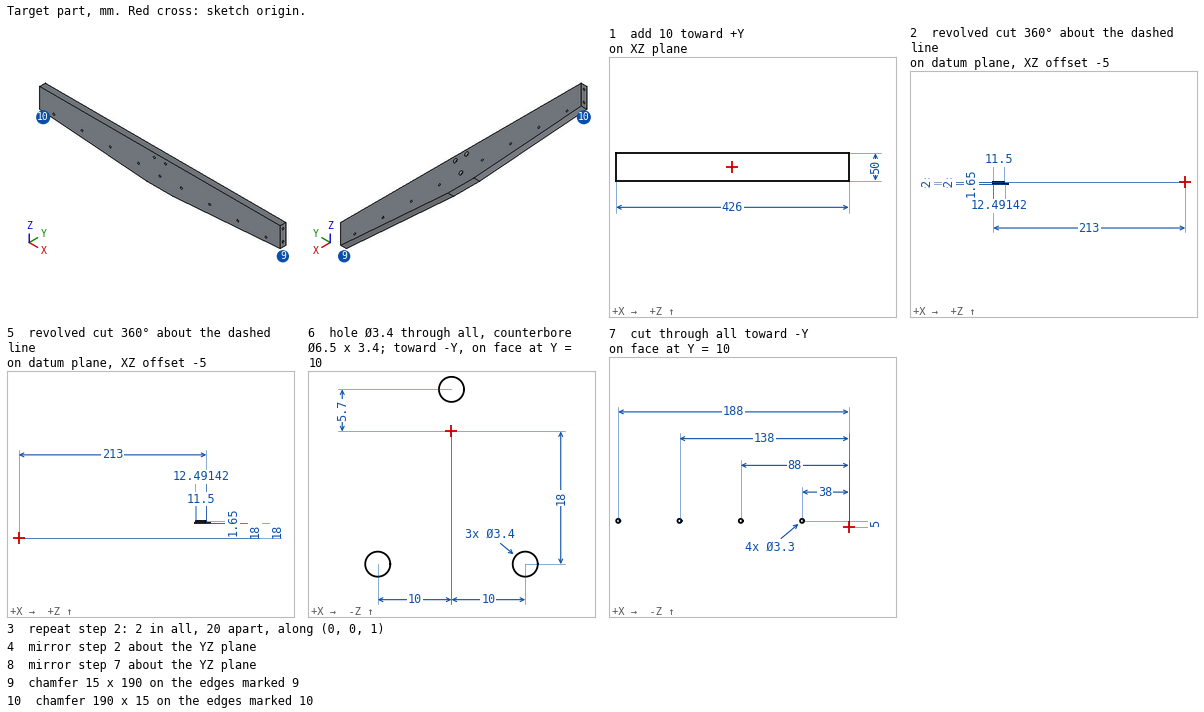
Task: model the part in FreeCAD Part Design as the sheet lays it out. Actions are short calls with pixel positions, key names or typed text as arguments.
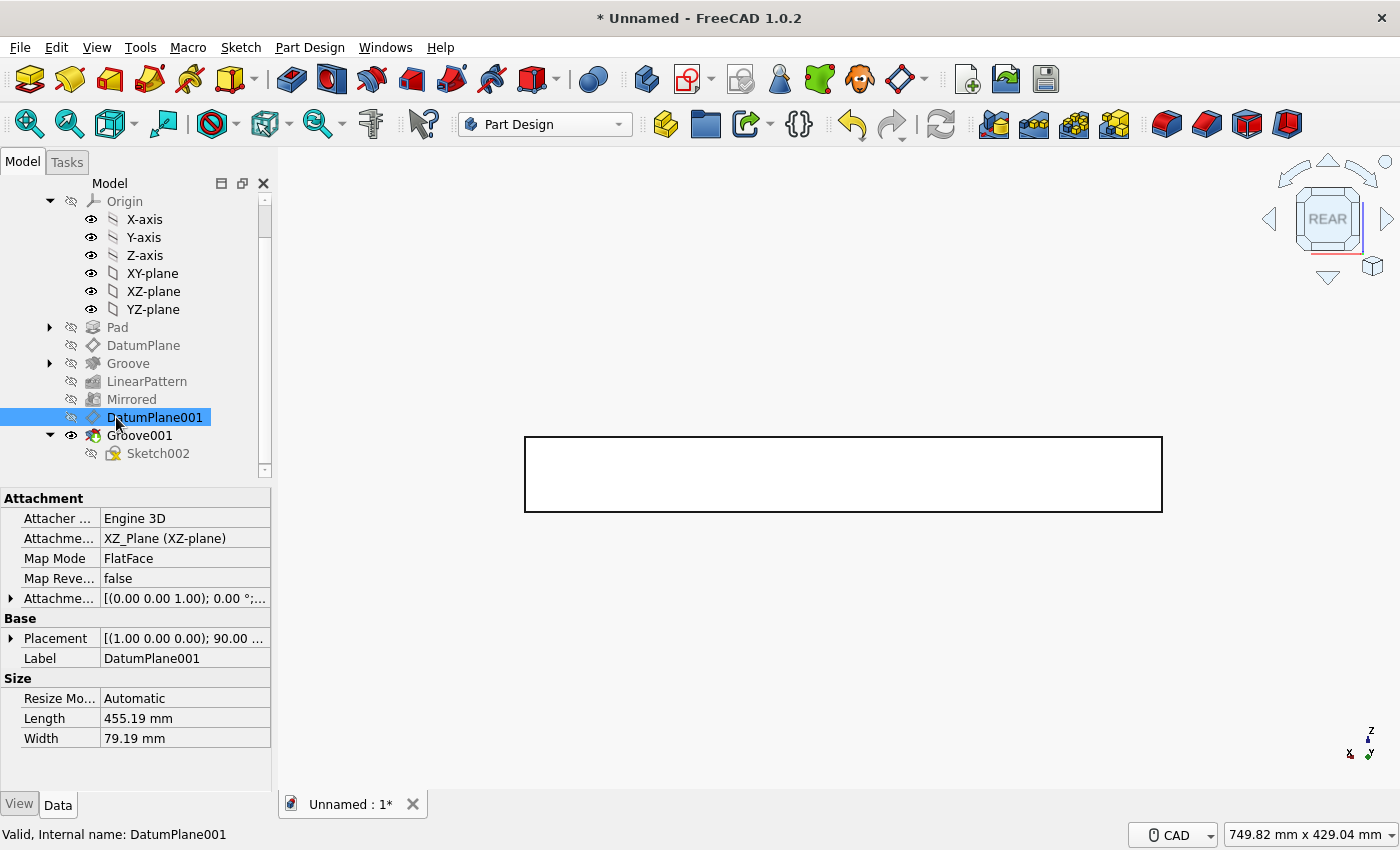
click(570, 474)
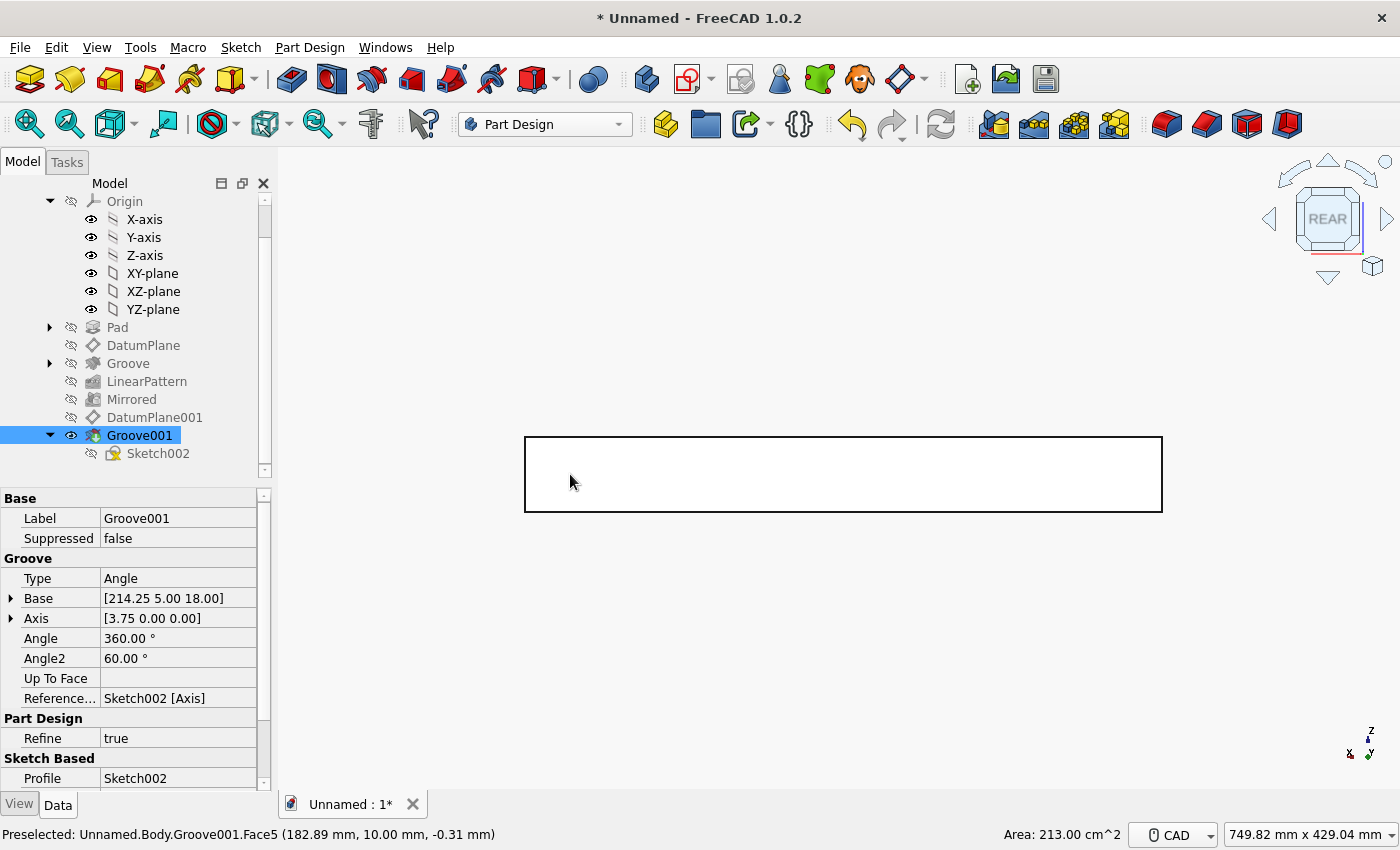
click(688, 80)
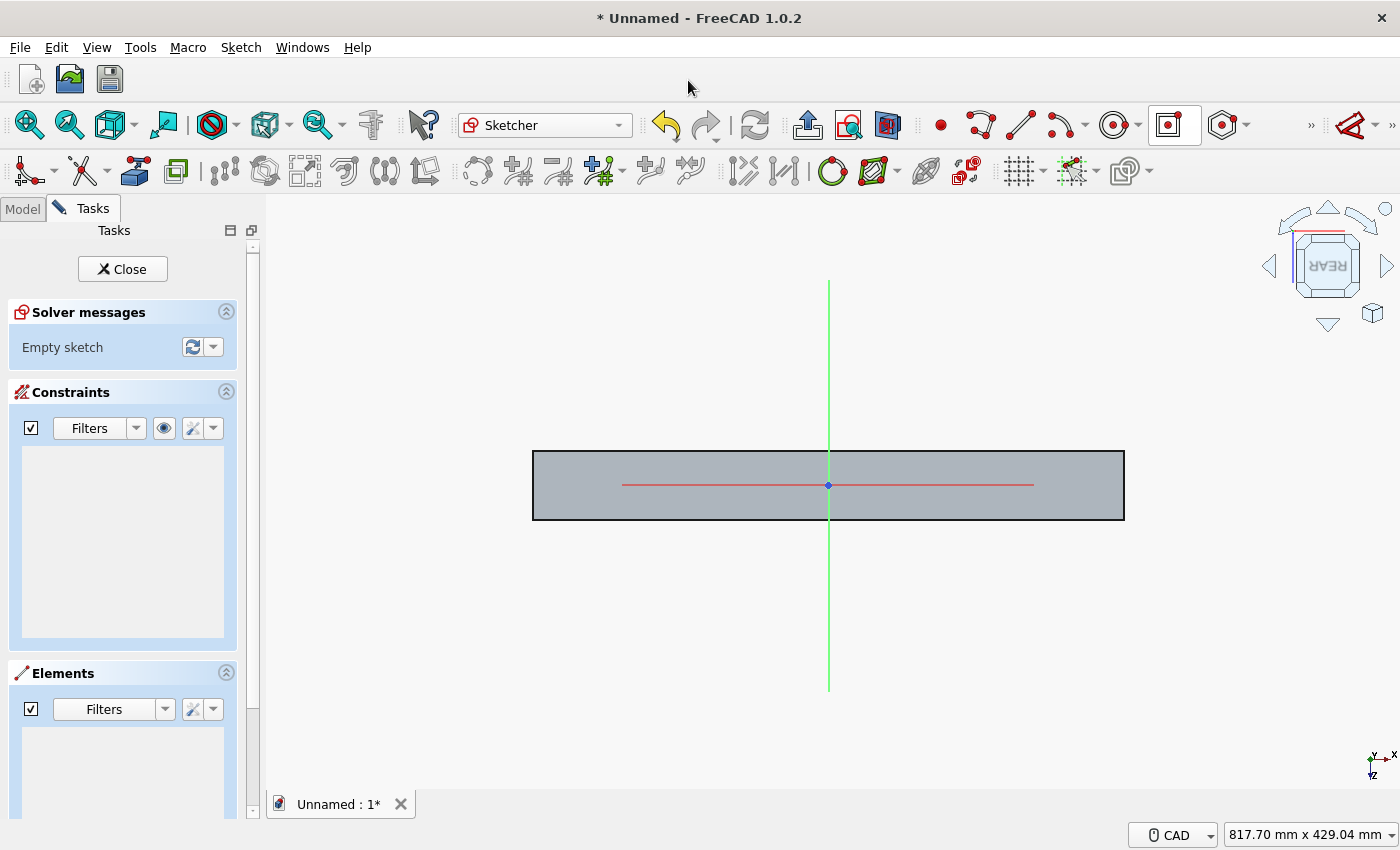
scroll(835, 494, up, 12)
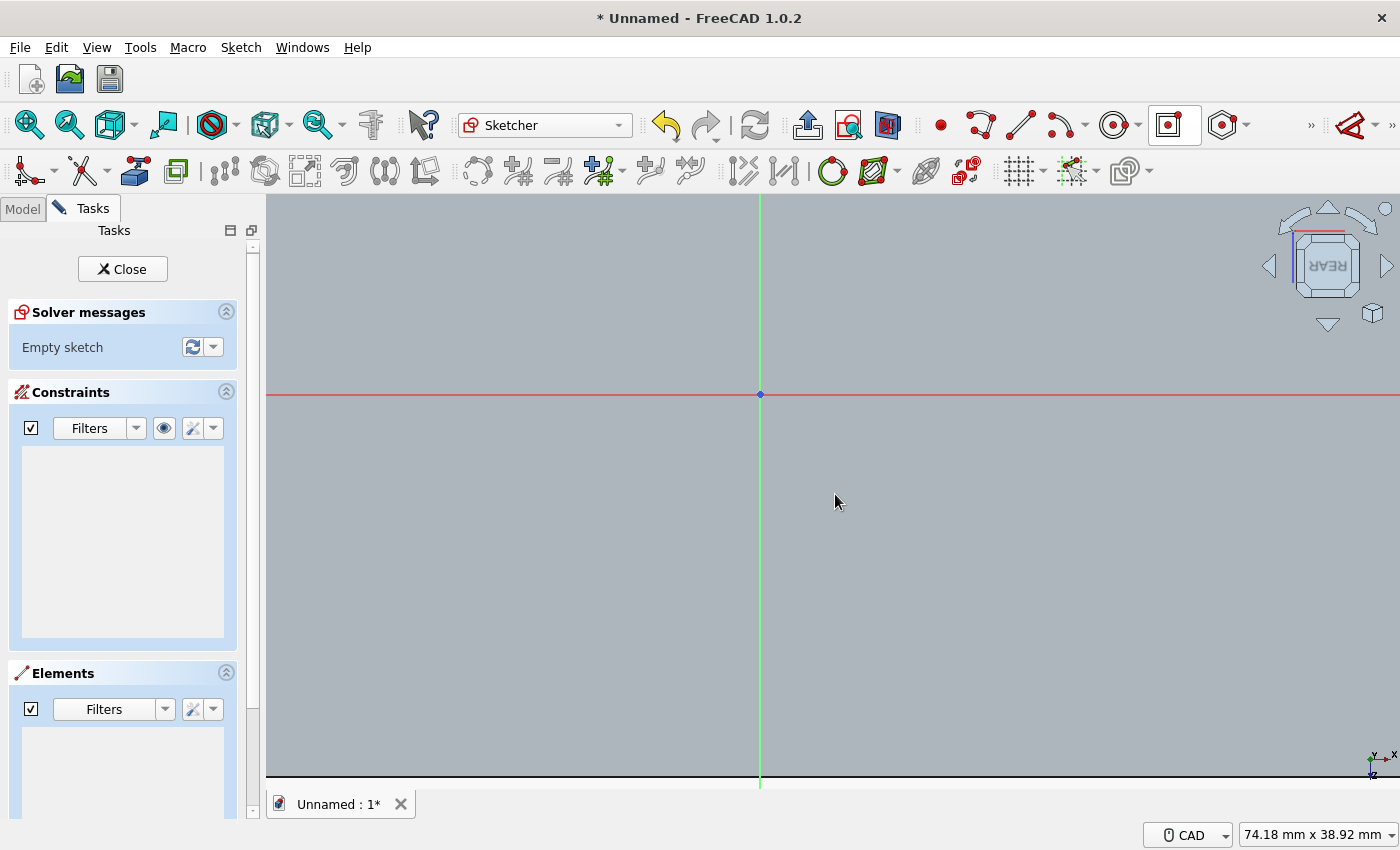
key(g)
key(c)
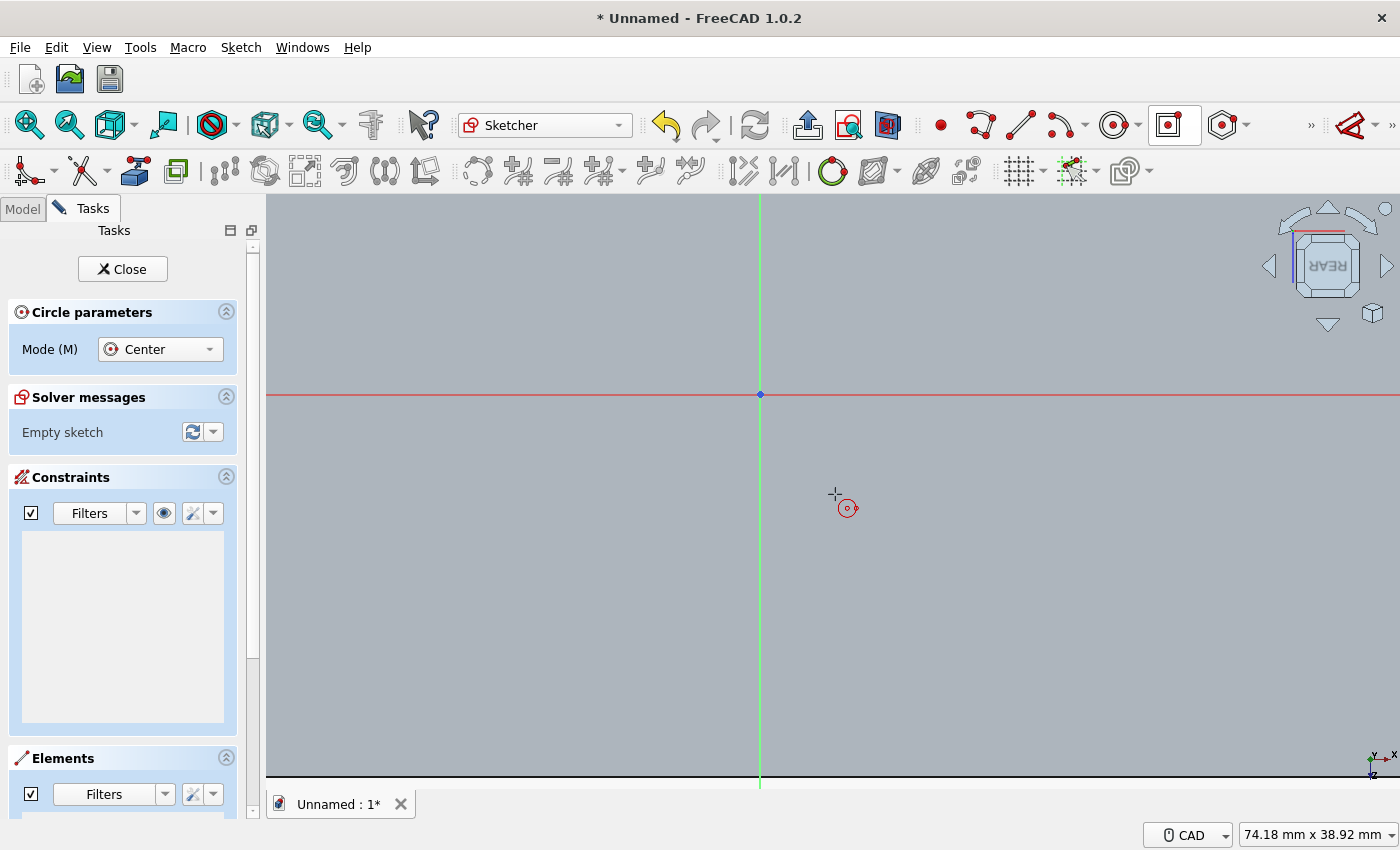
click(913, 670)
move(931, 651)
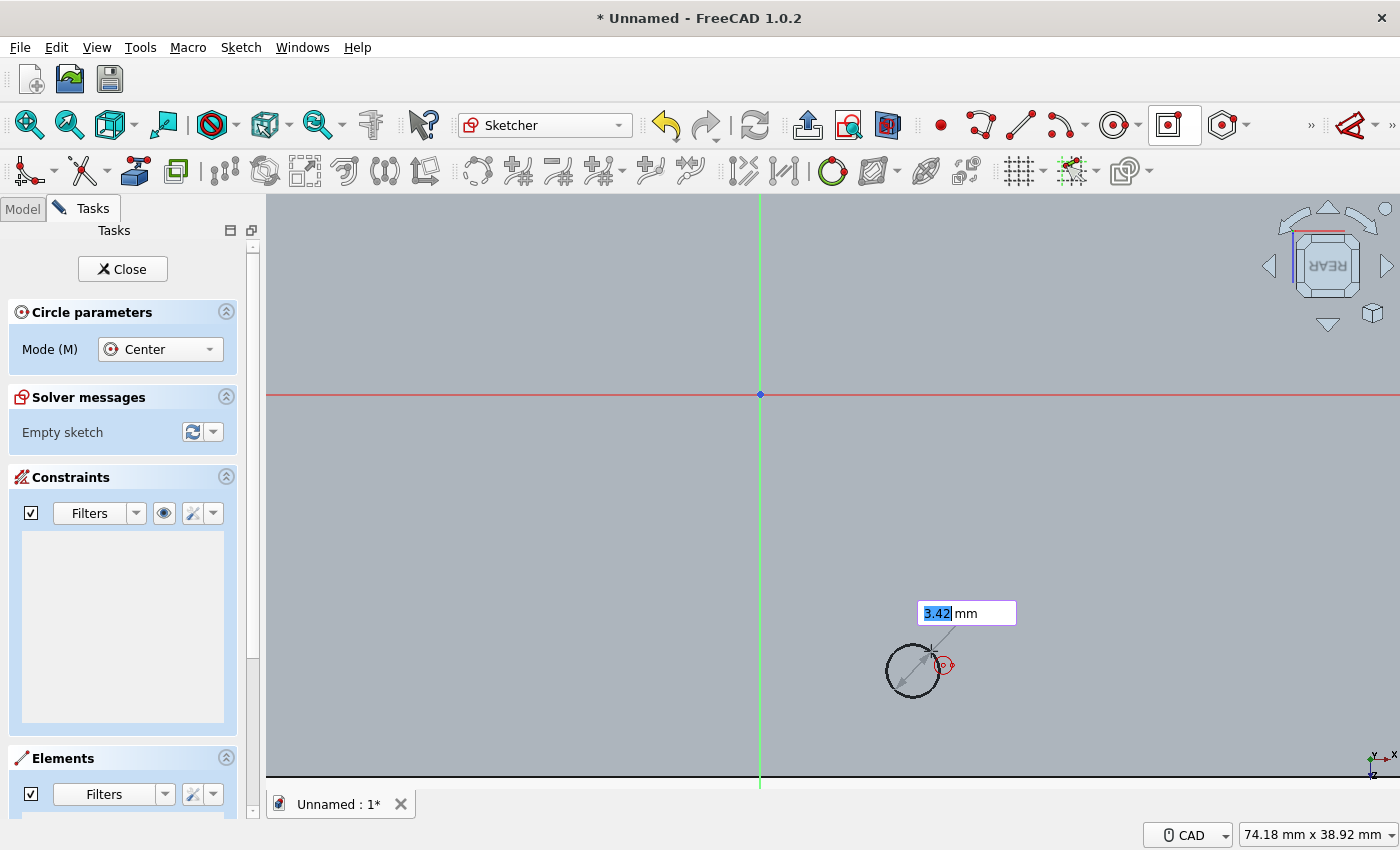
text(3.4)
key(Return)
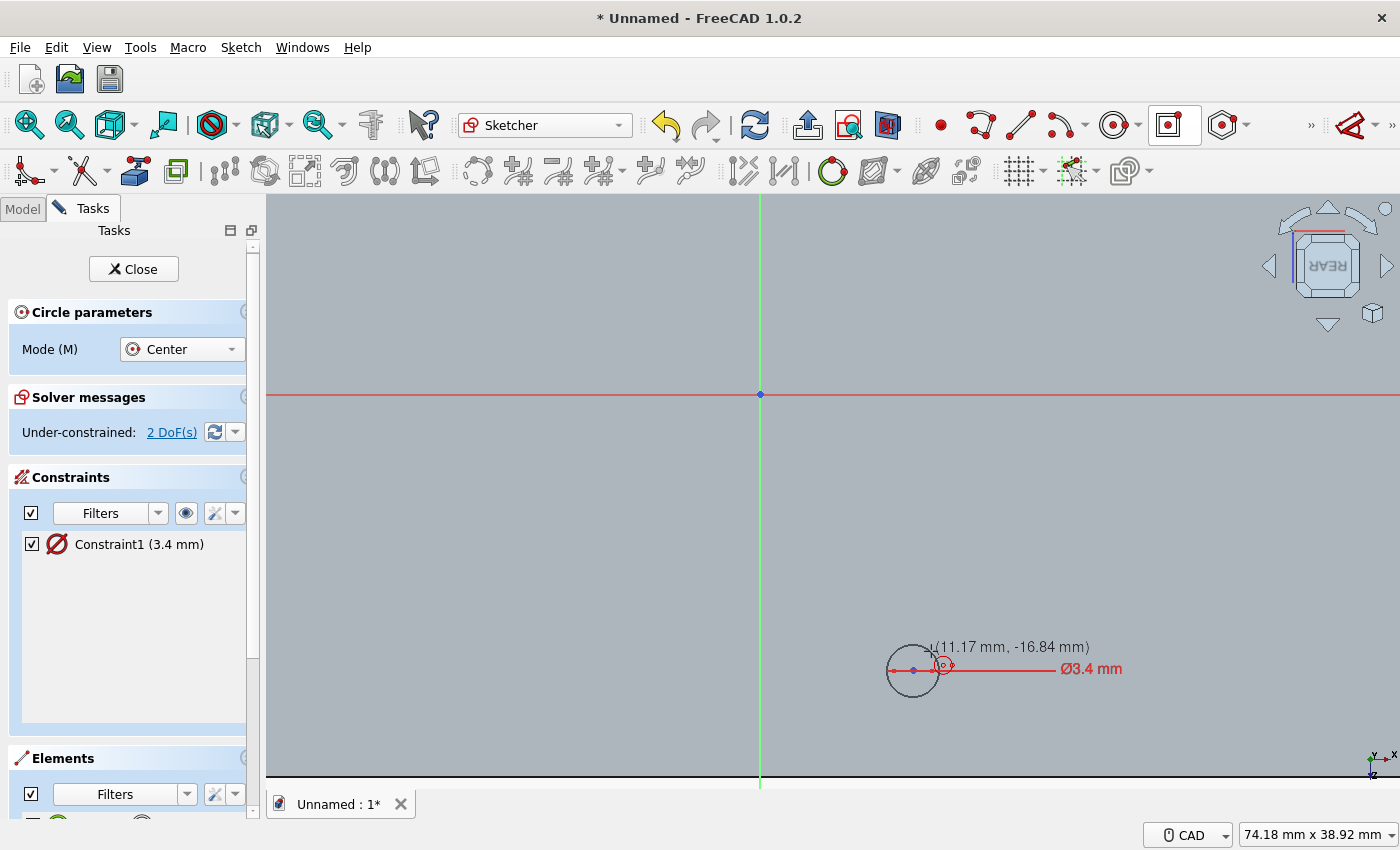
click(607, 670)
move(626, 651)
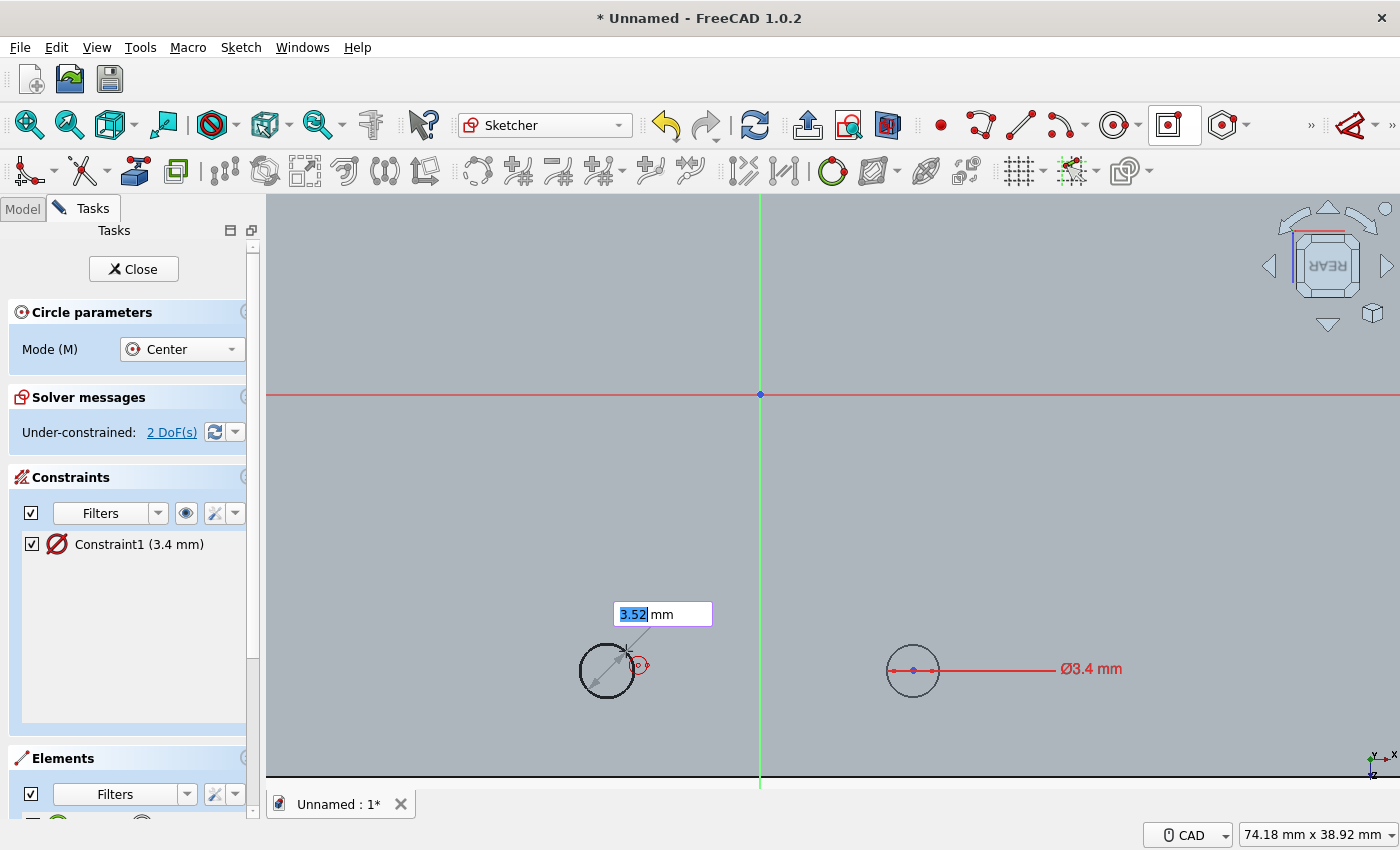
text(3.4)
key(Return)